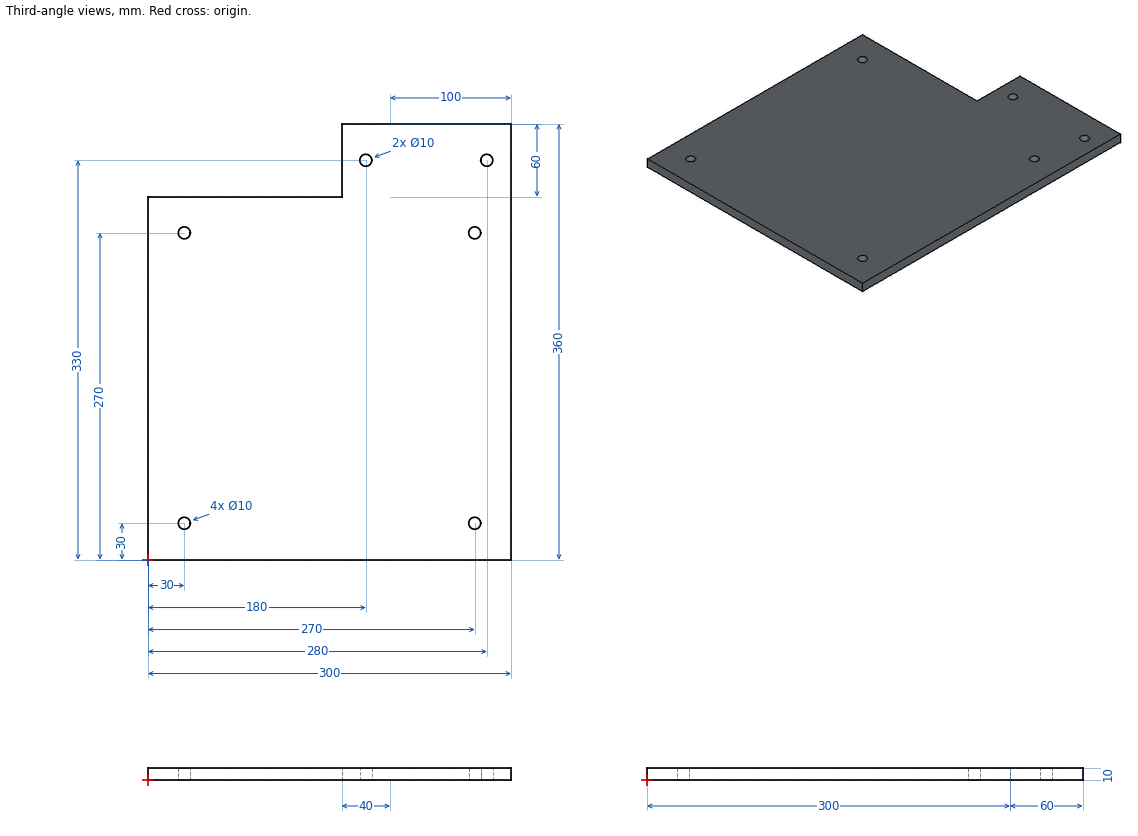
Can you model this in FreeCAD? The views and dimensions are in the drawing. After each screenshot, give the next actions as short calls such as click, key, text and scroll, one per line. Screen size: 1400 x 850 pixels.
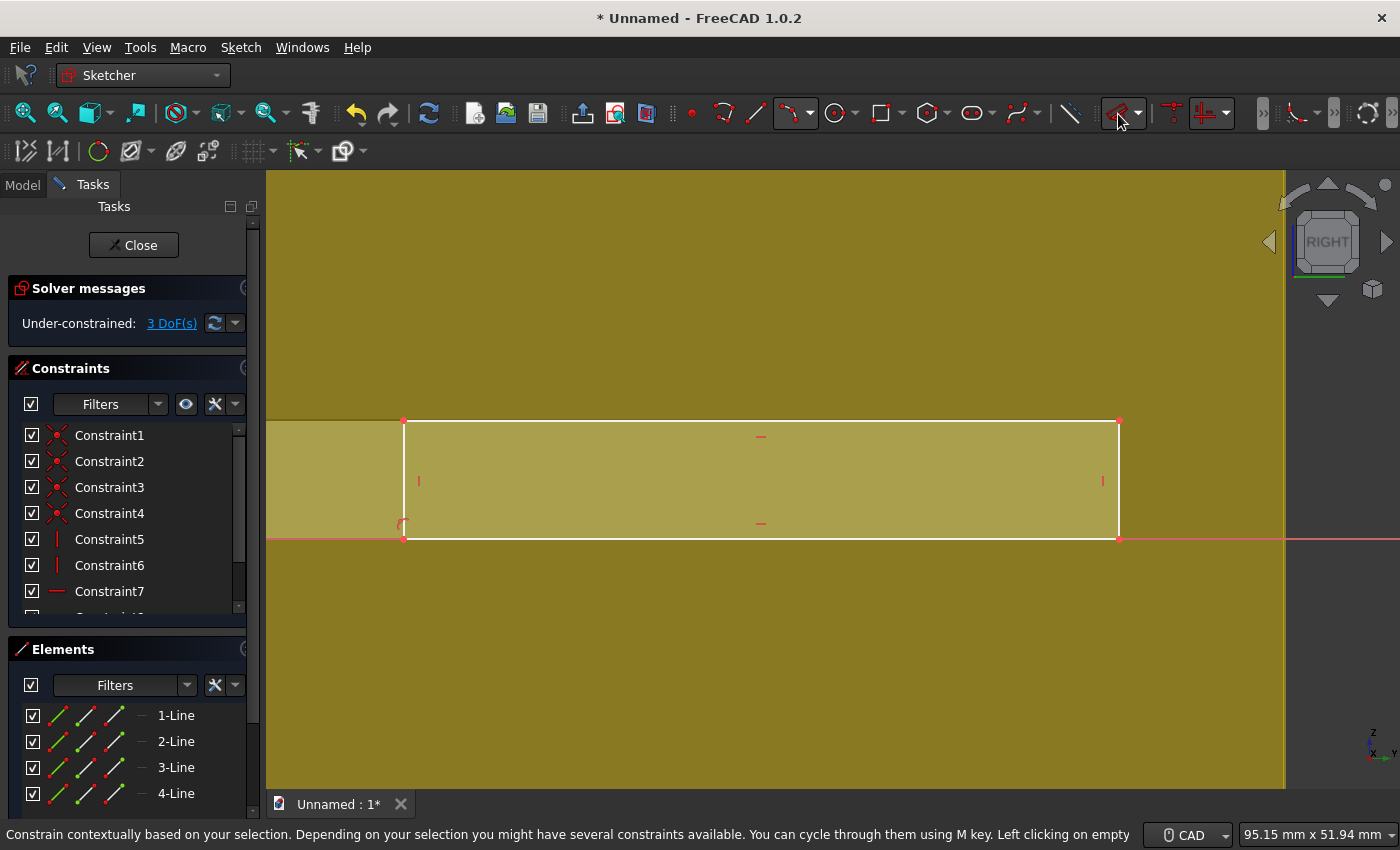
click(404, 456)
click(370, 480)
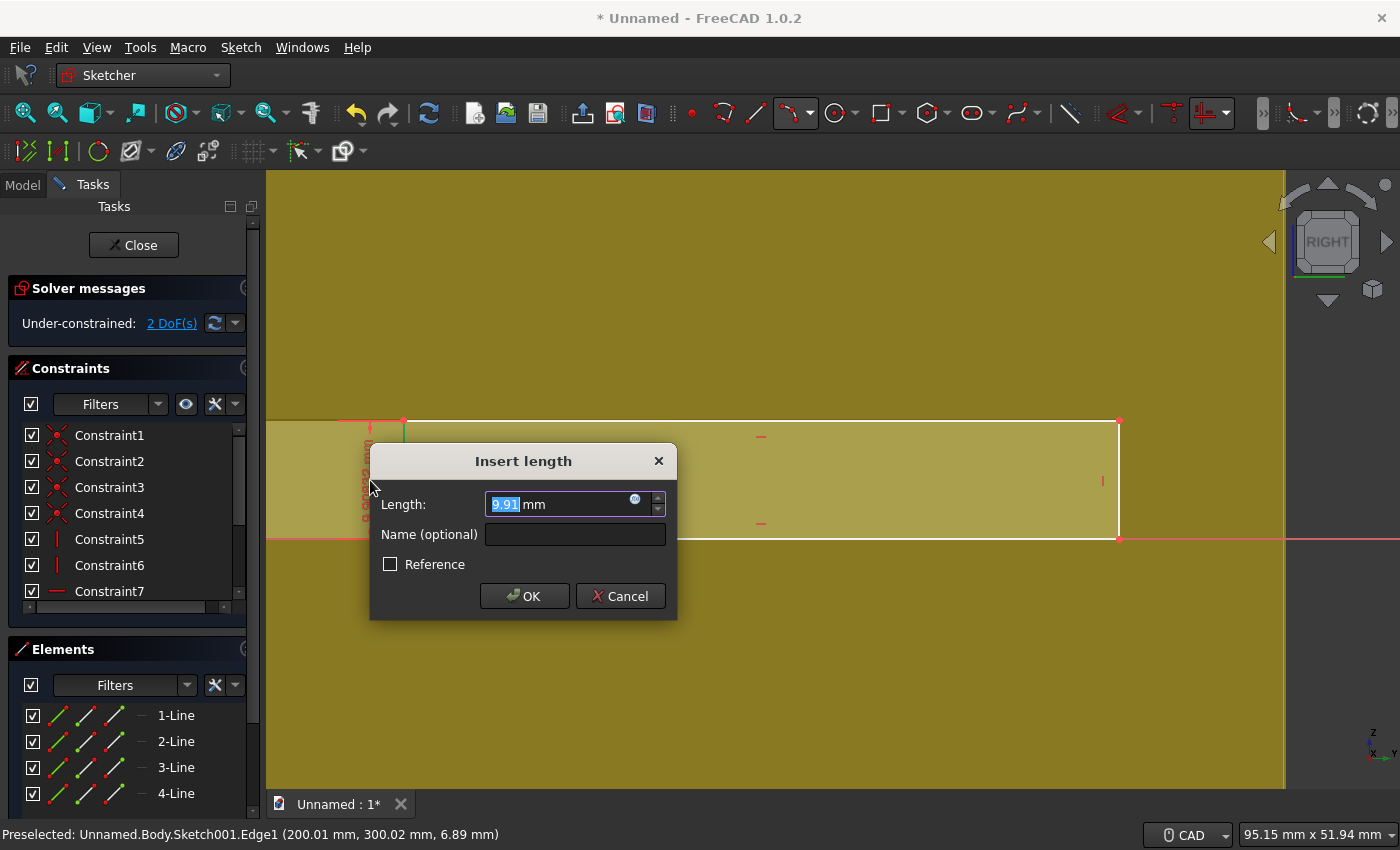
text(10)
key(Return)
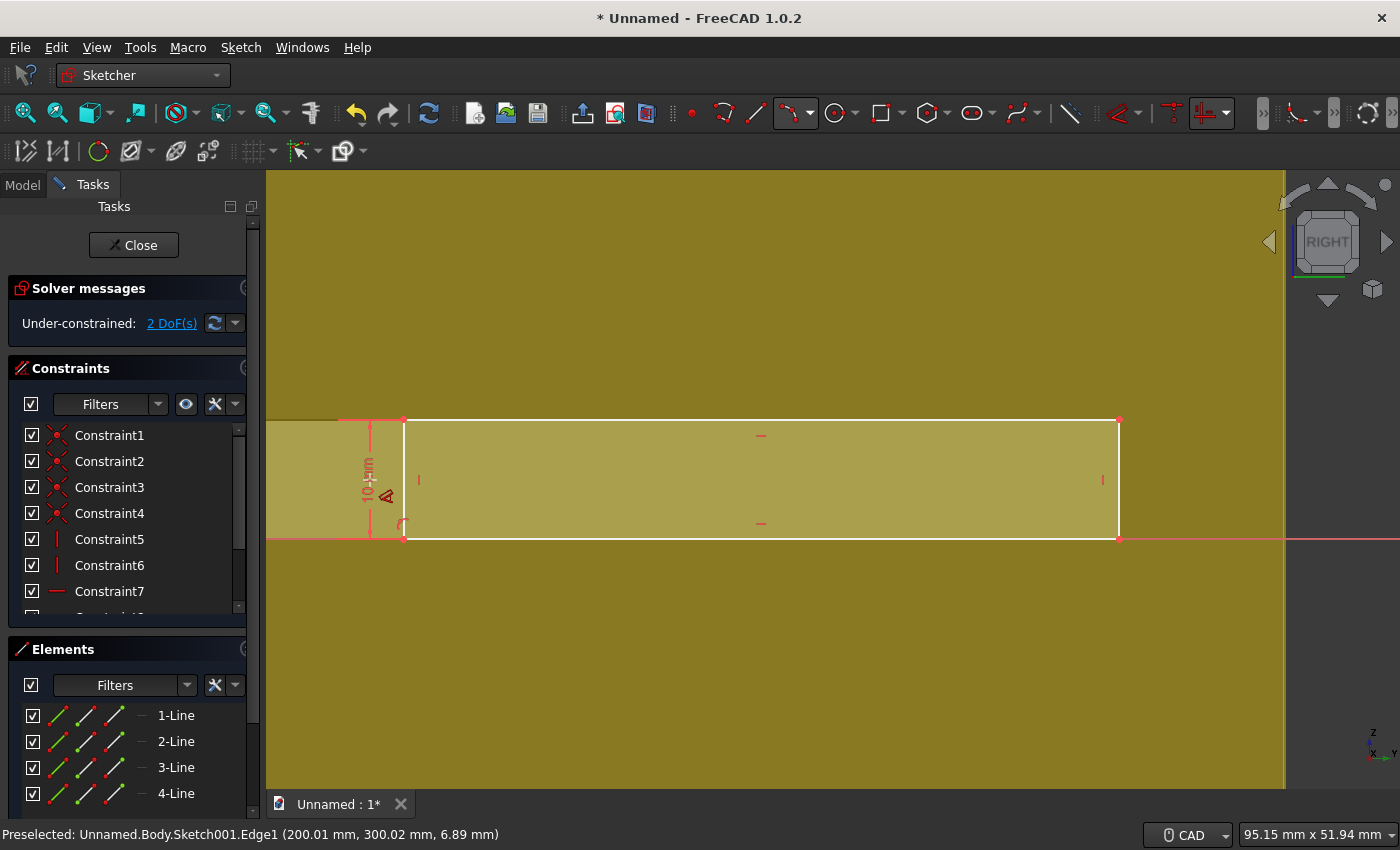
click(618, 539)
click(761, 573)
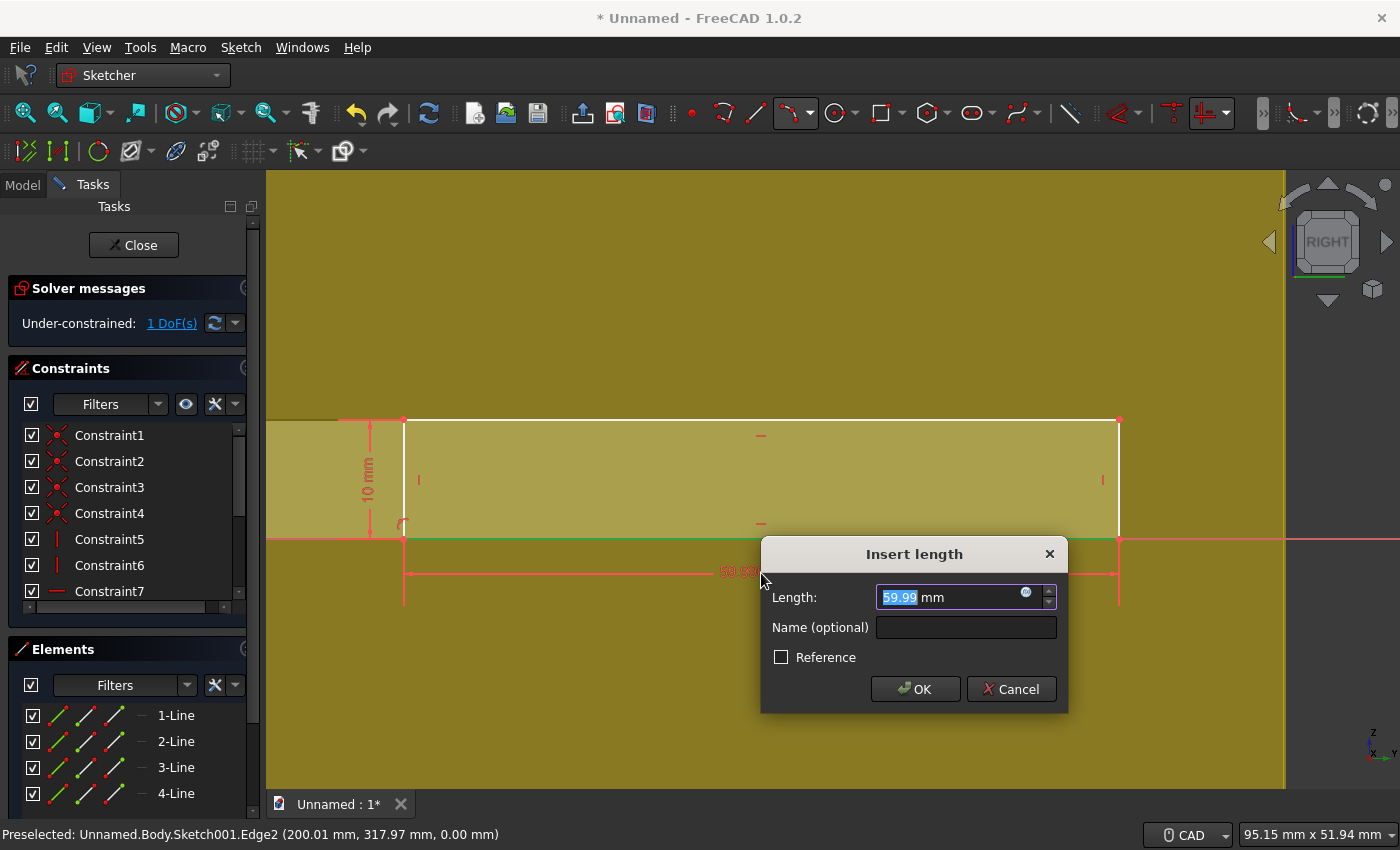
text(60)
key(Return)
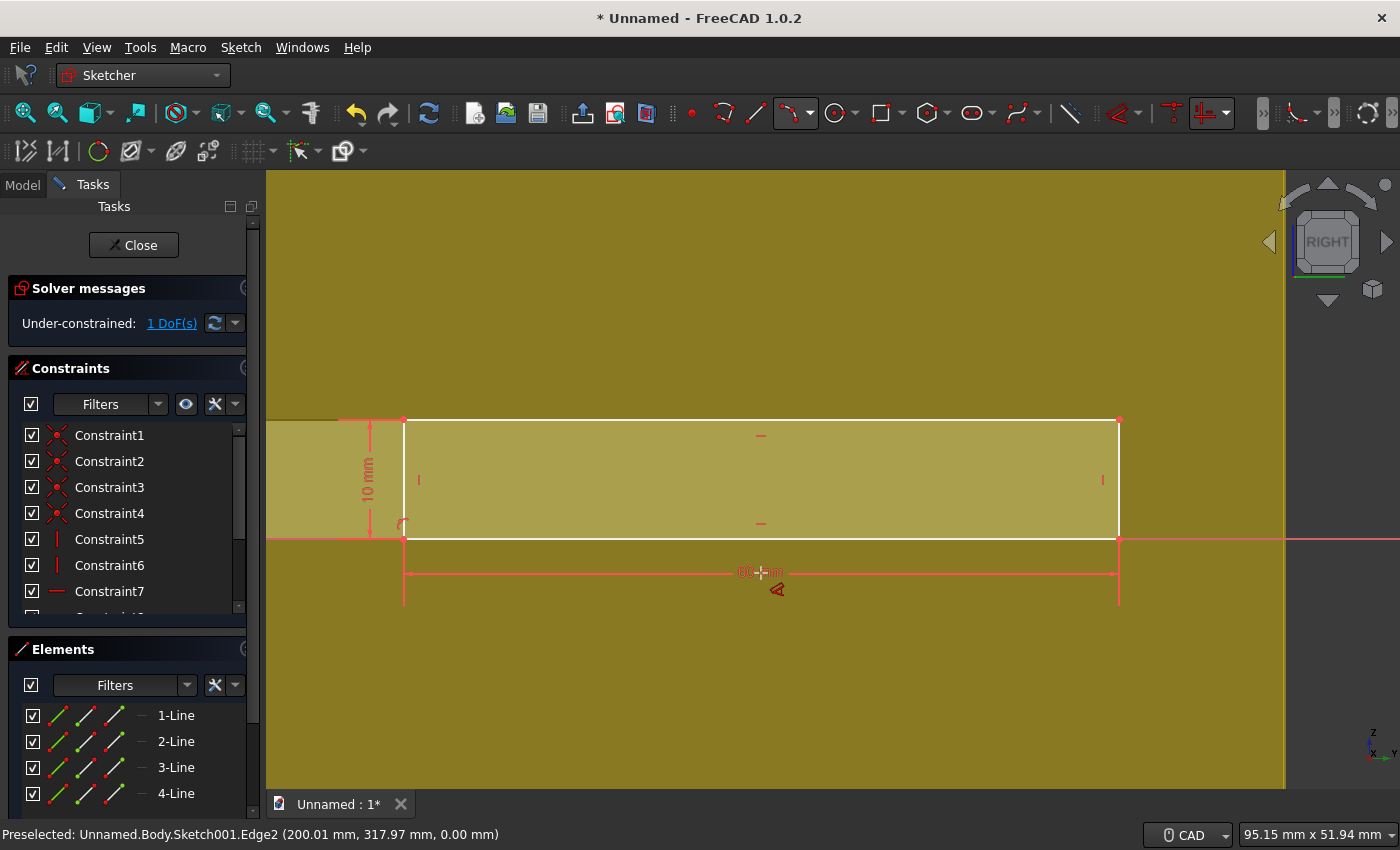
click(404, 420)
click(349, 573)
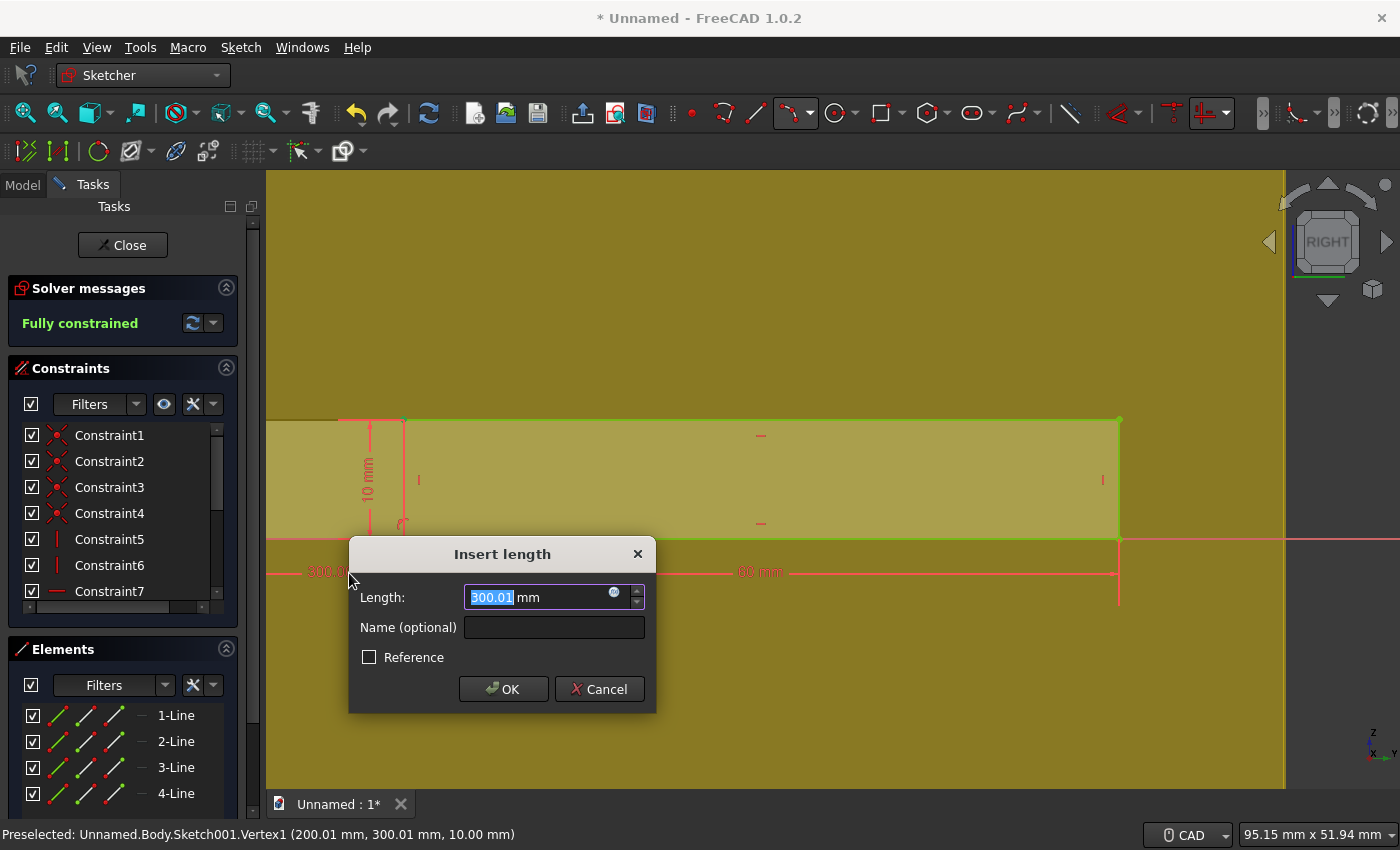
text(300)
key(Return)
key(Escape)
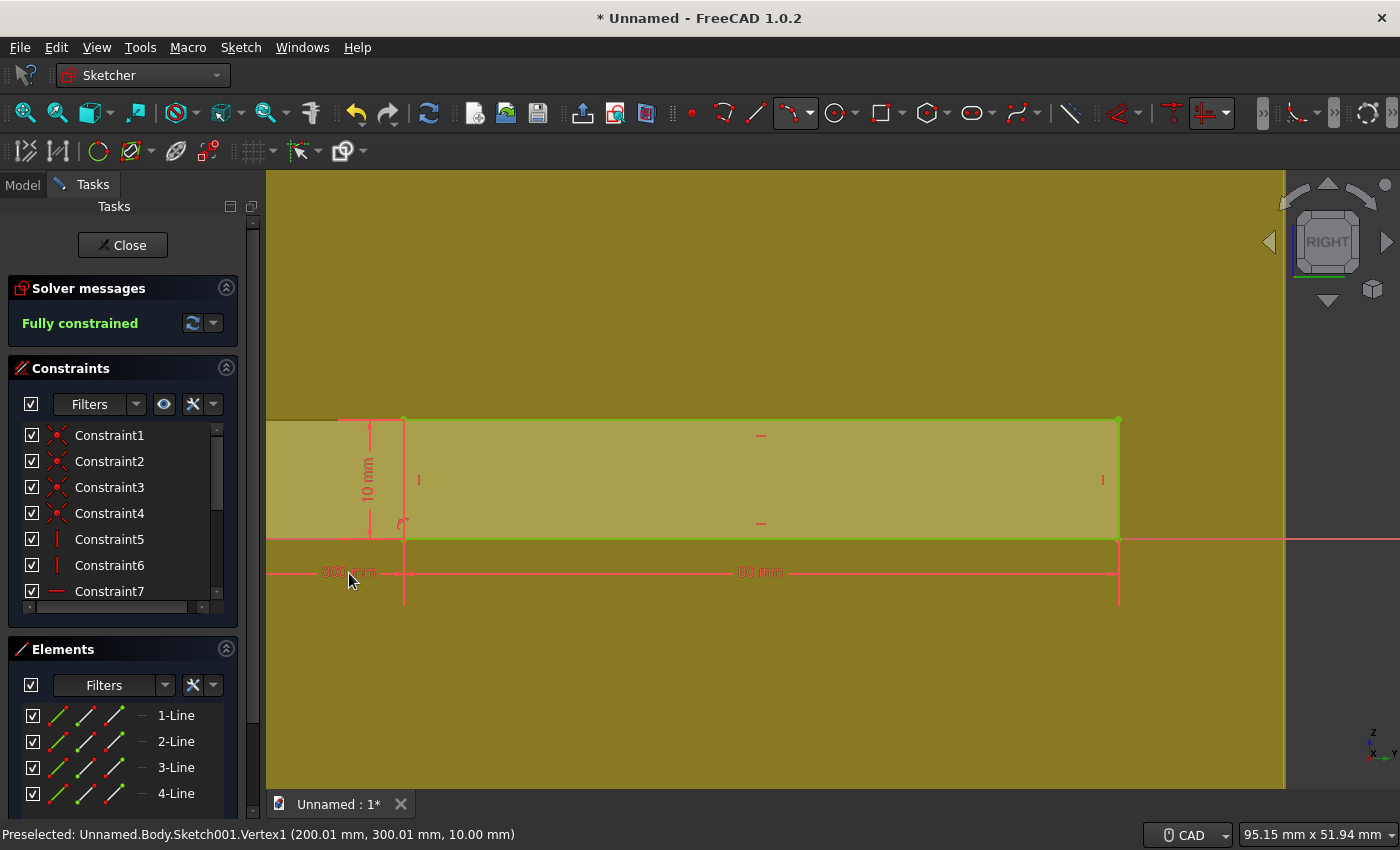
click(123, 245)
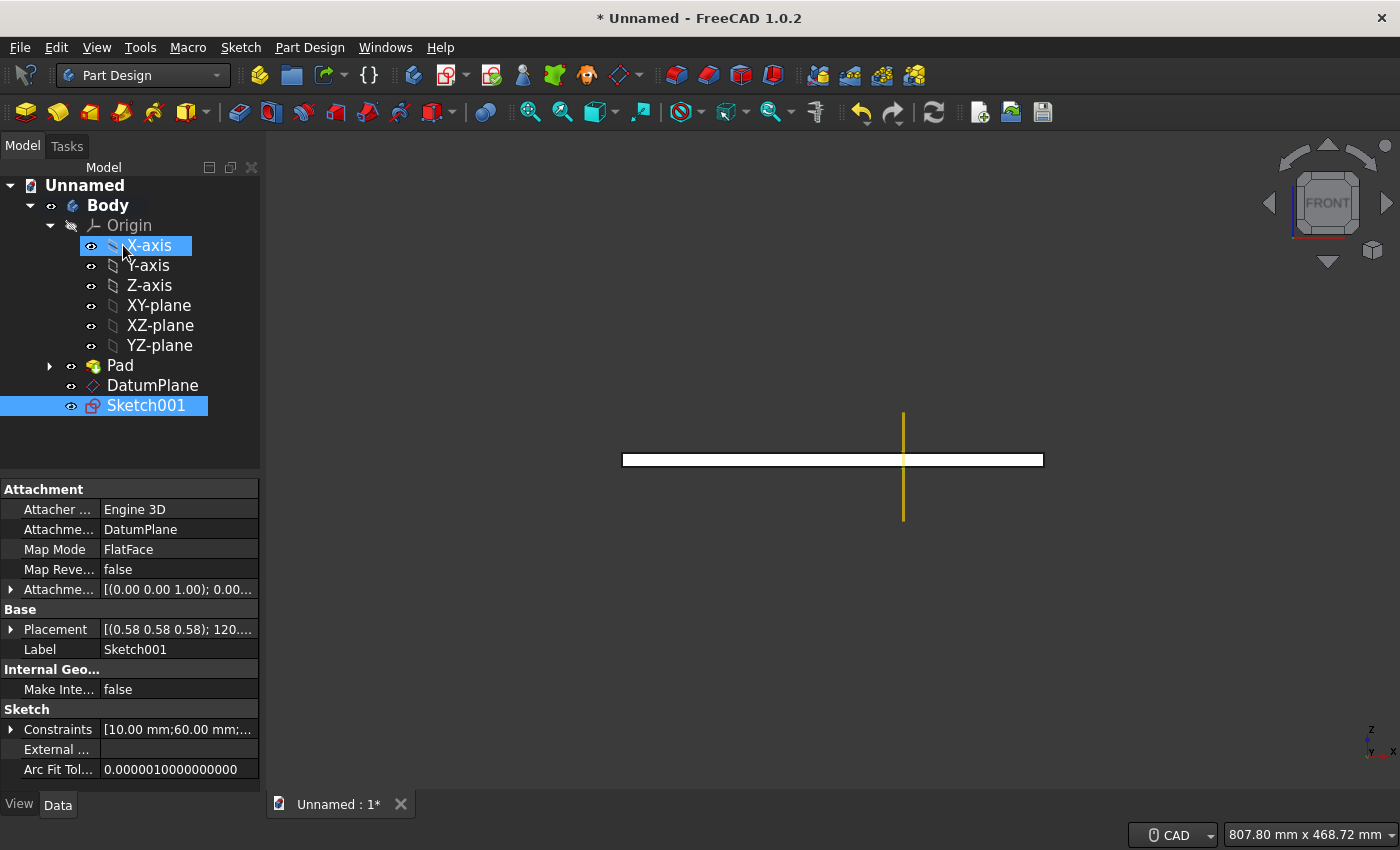
click(26, 112)